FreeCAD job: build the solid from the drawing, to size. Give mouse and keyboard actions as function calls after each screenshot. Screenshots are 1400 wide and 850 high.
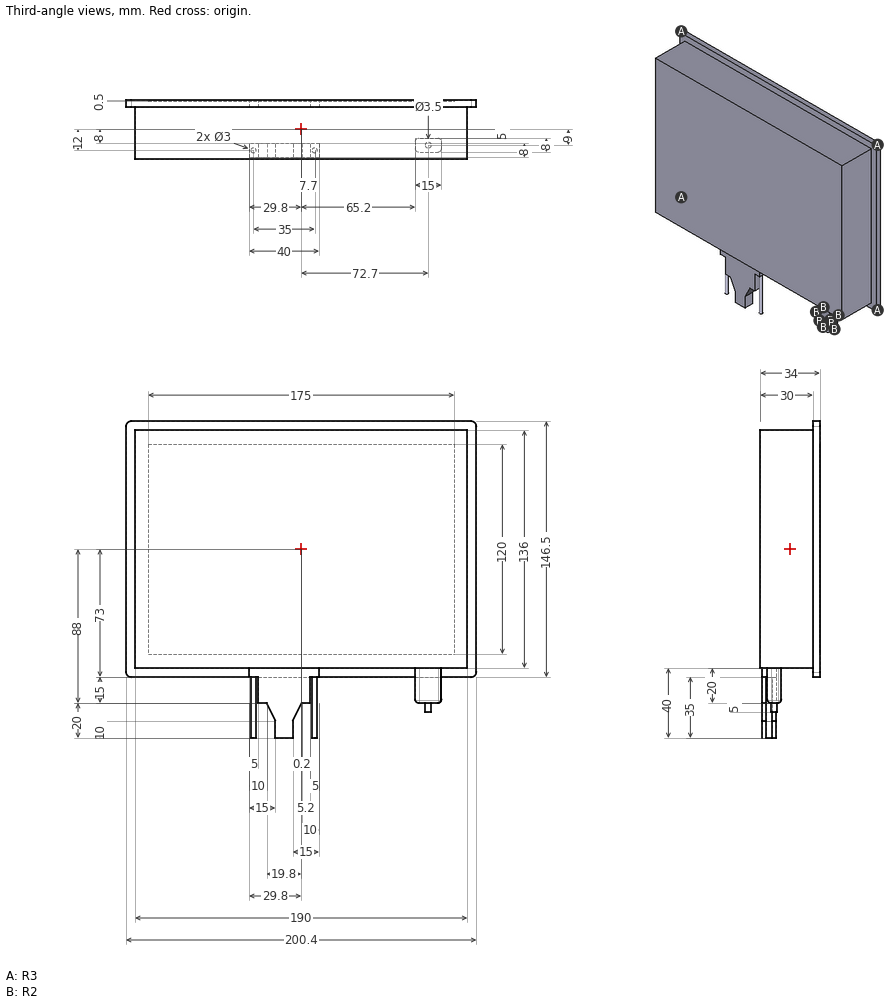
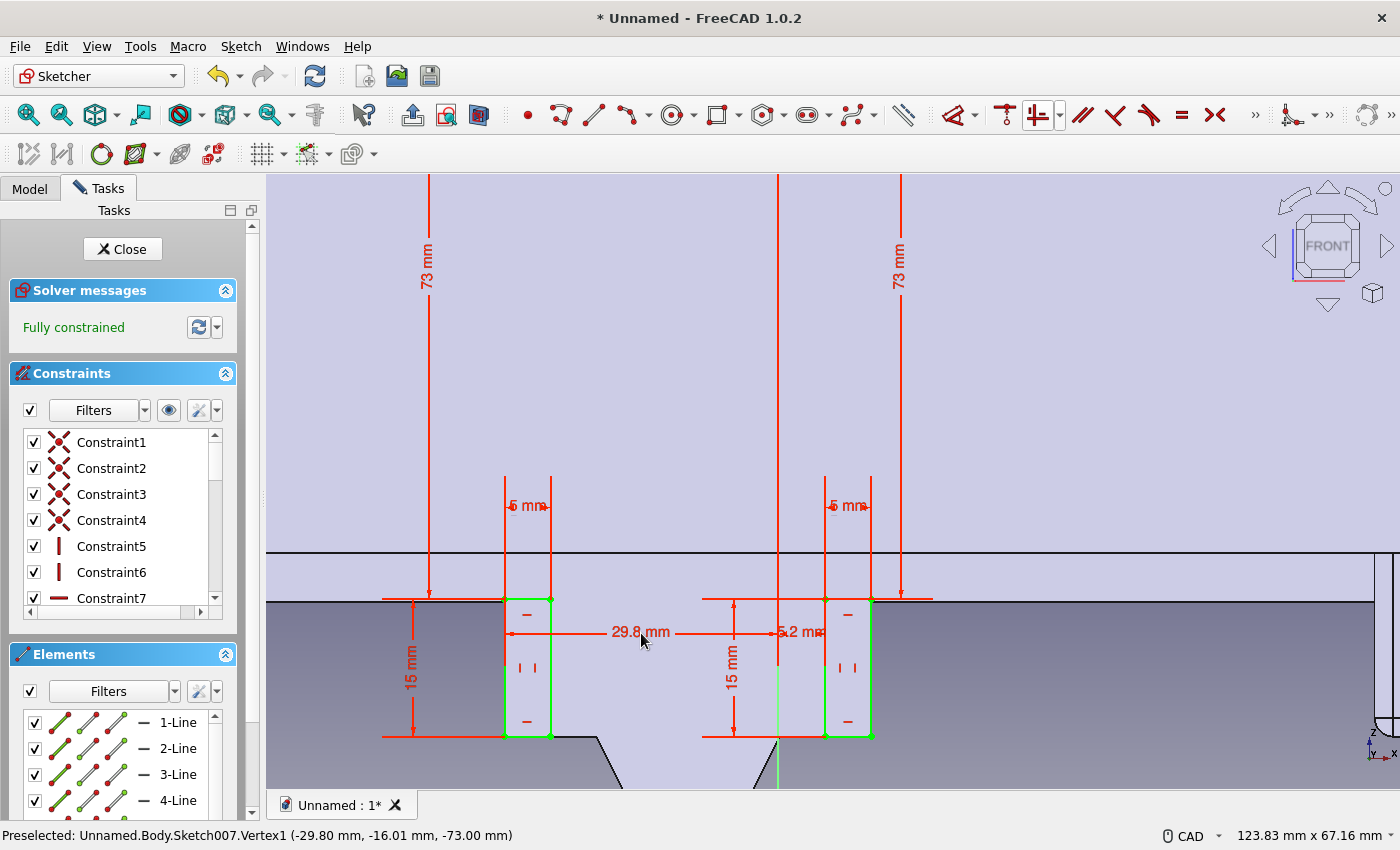
click(123, 249)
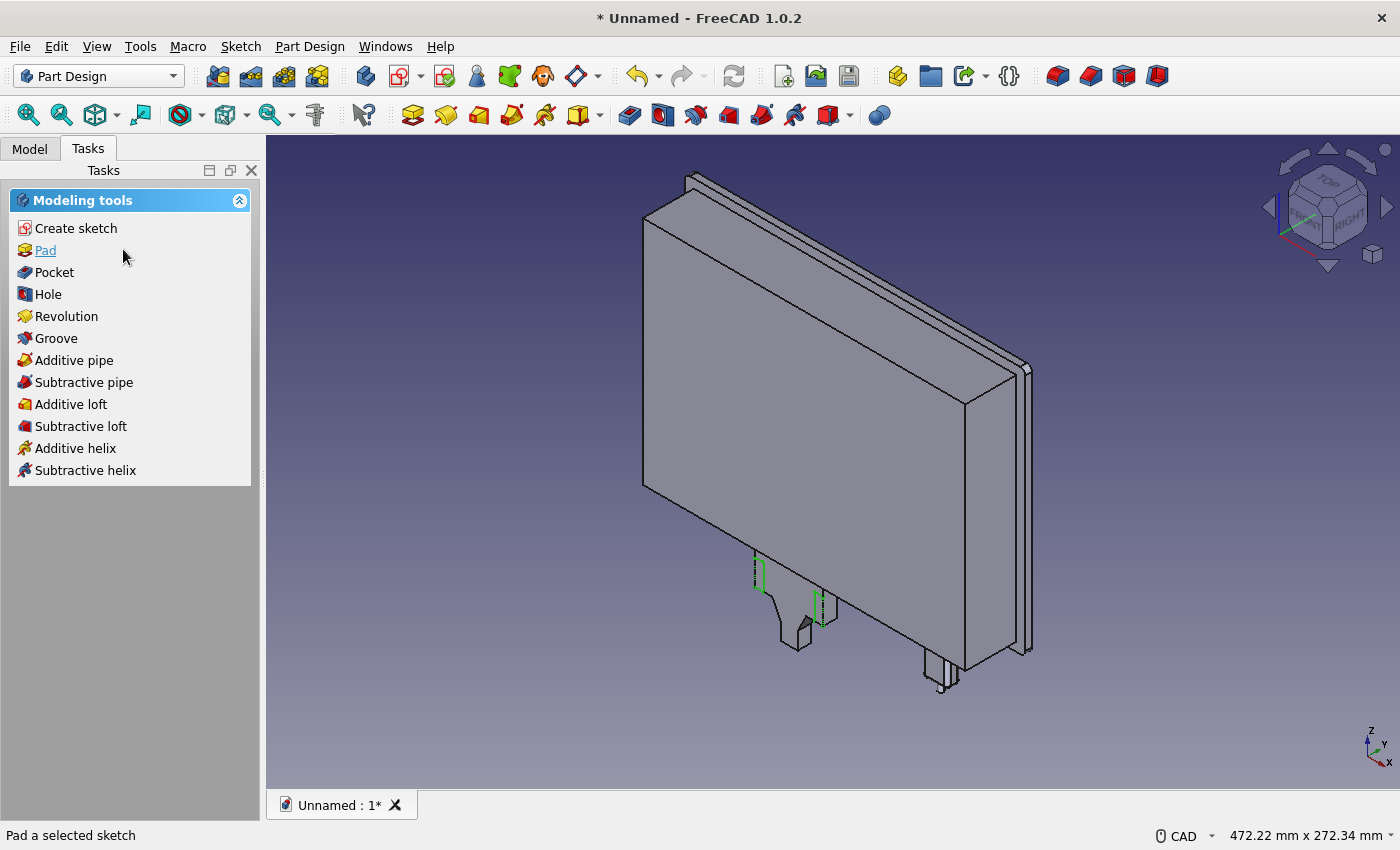
click(630, 116)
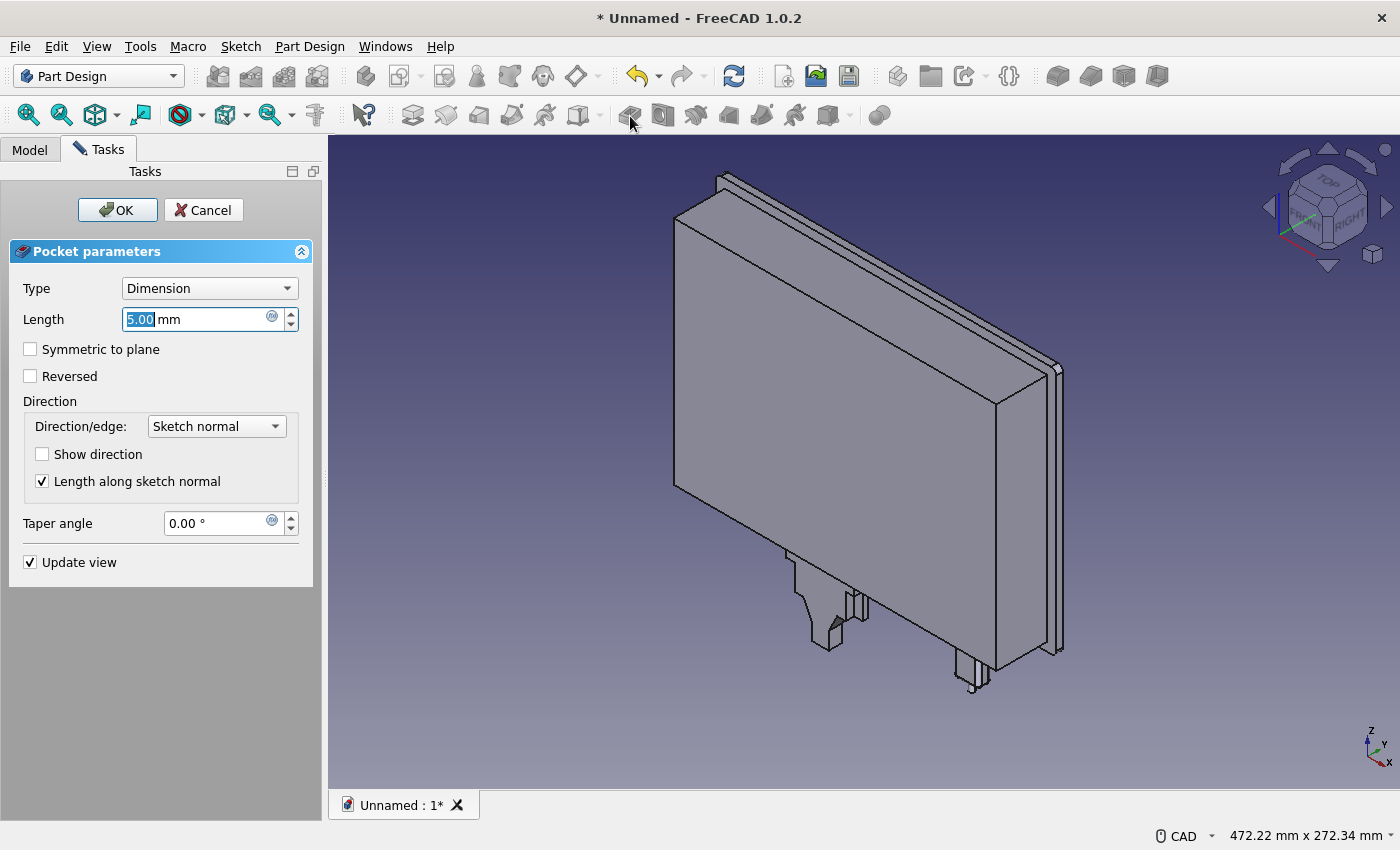
click(210, 288)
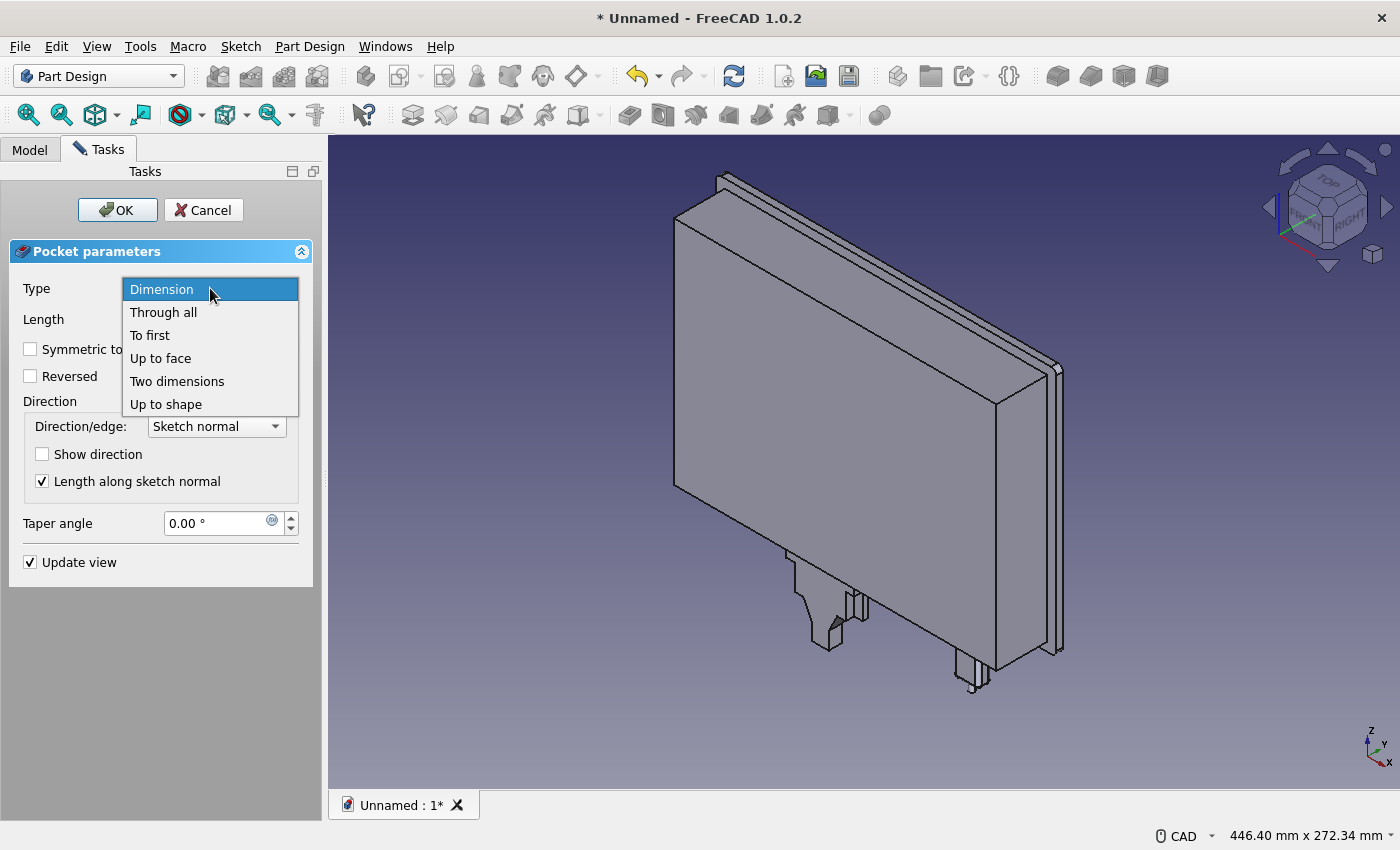
click(208, 312)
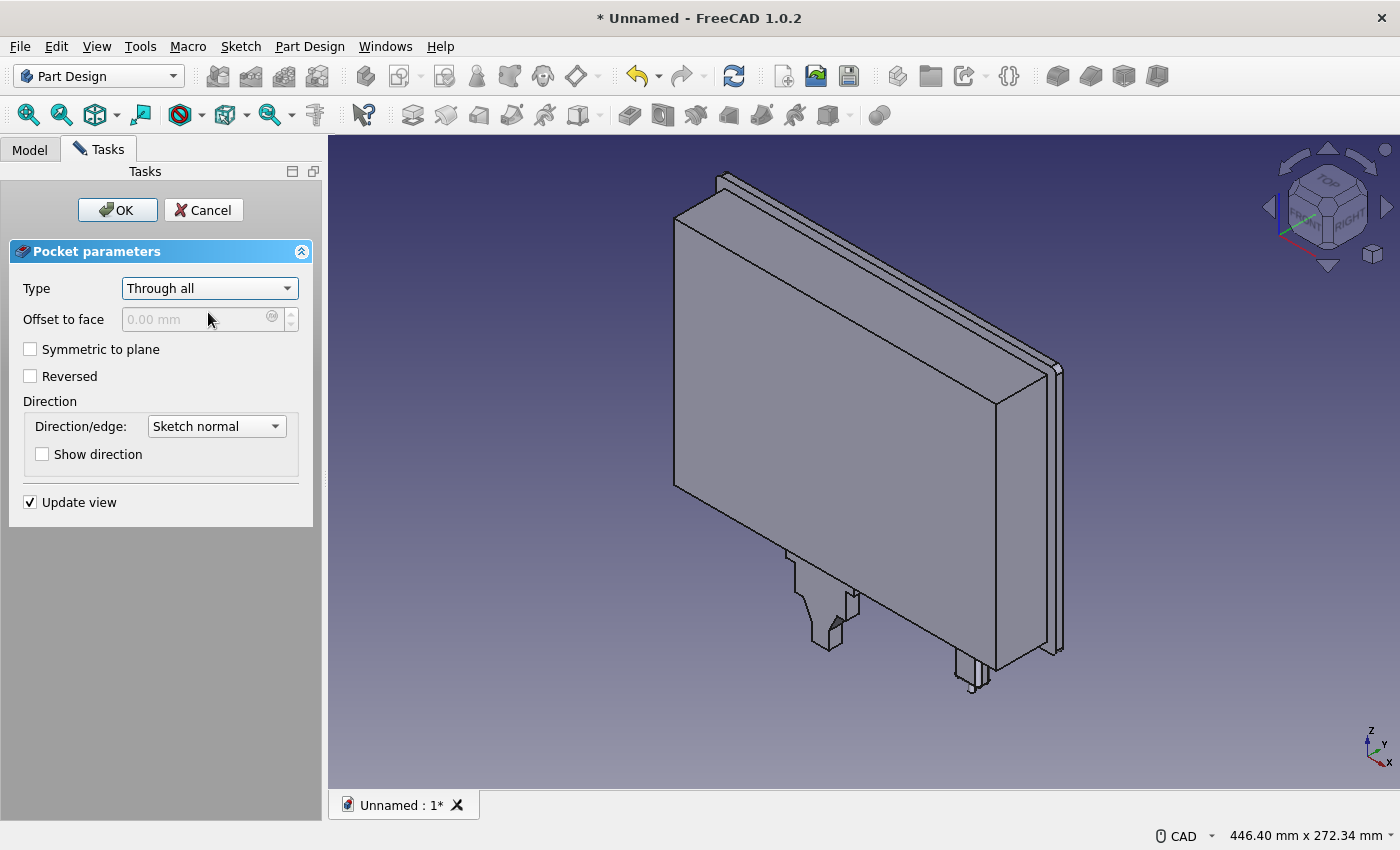
click(118, 210)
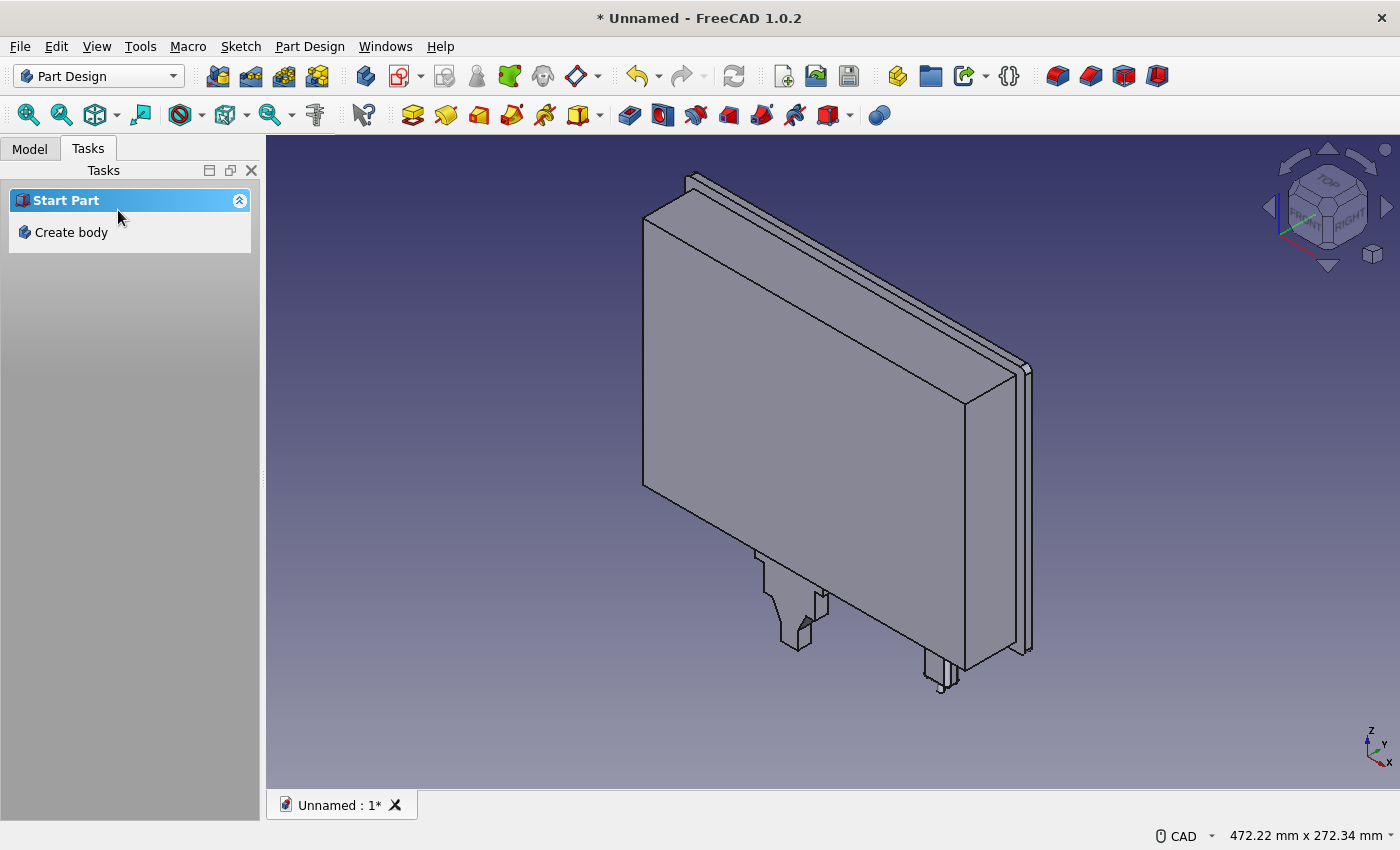
key(5)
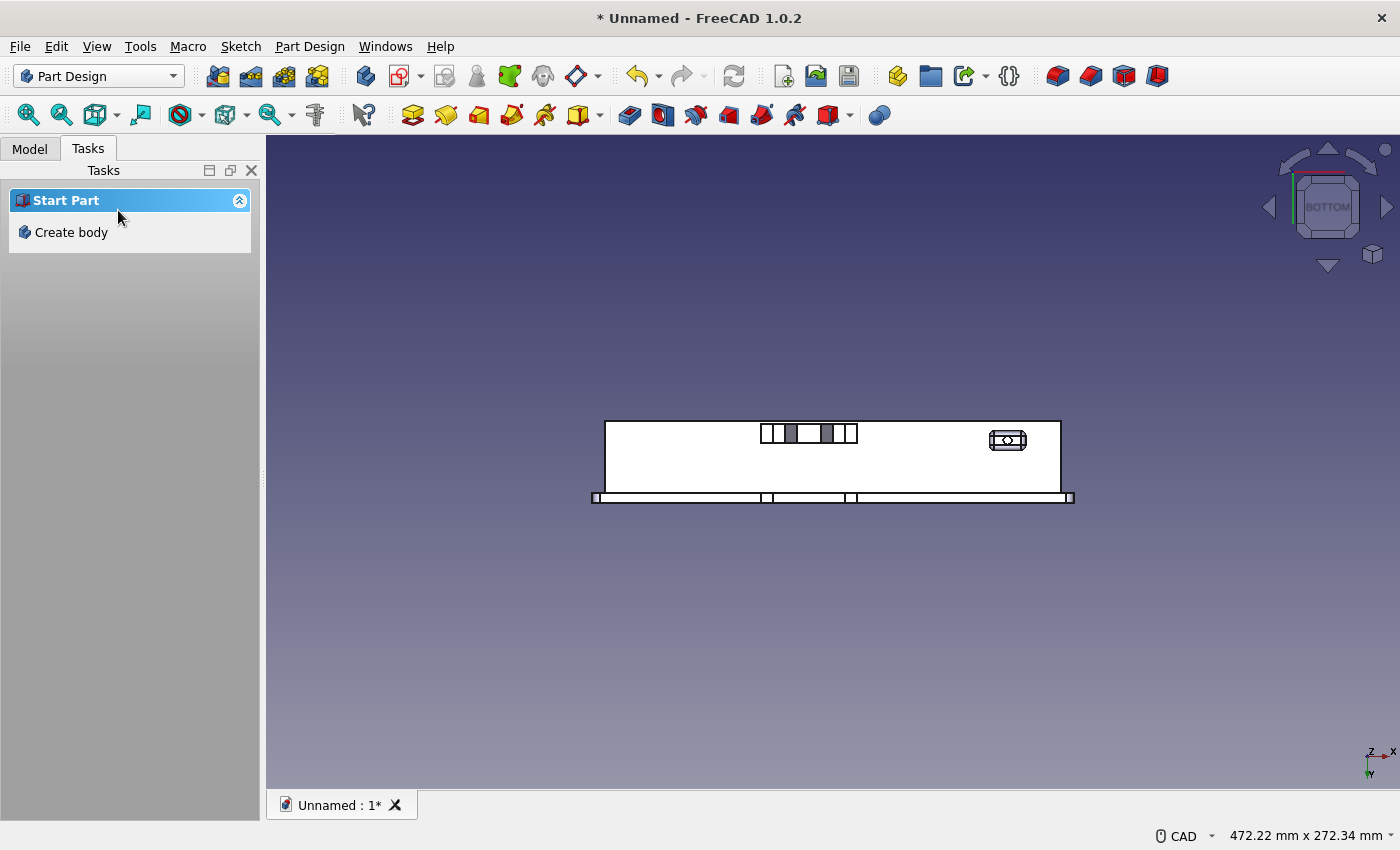
click(29, 116)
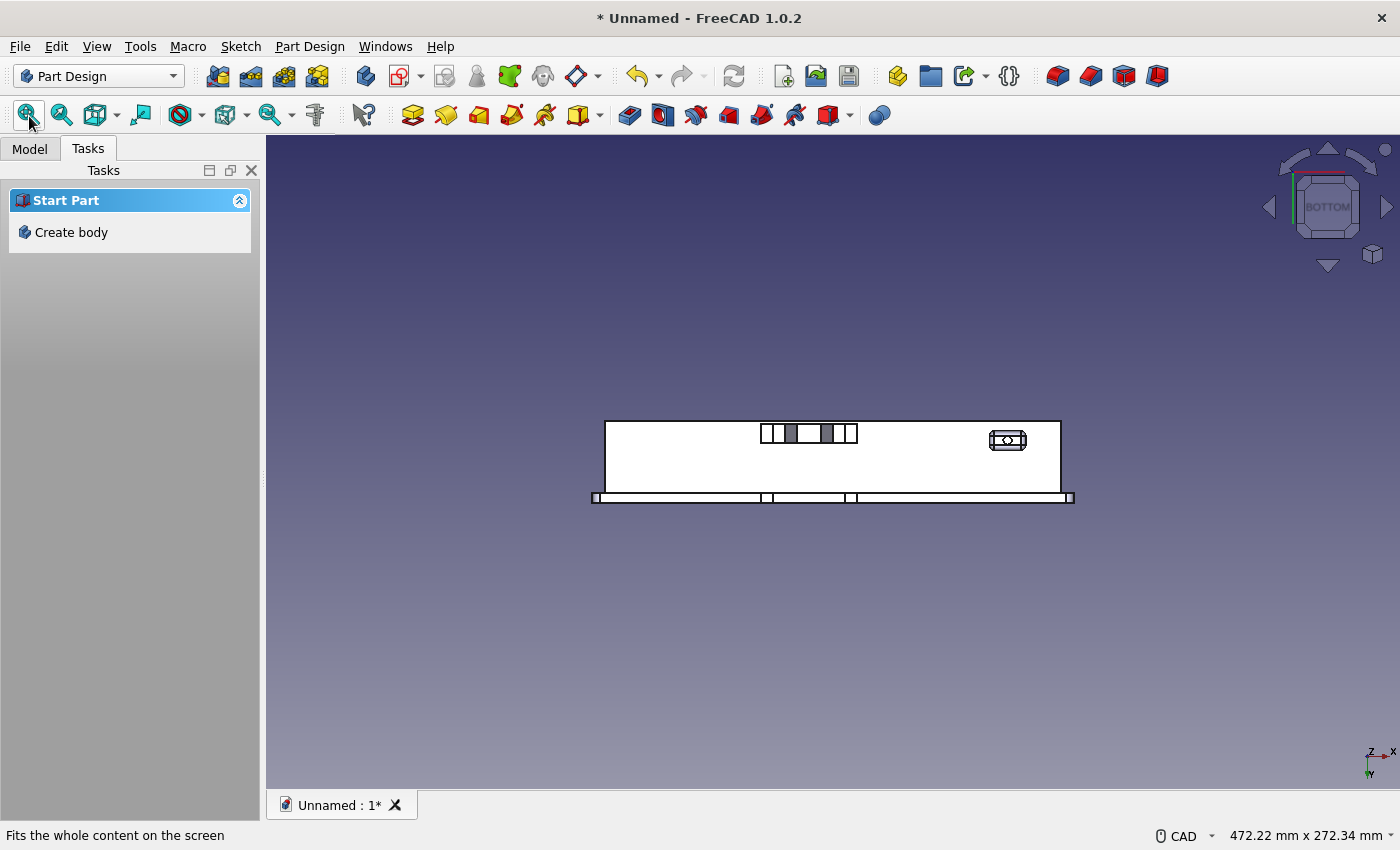
scroll(767, 435, up, 4)